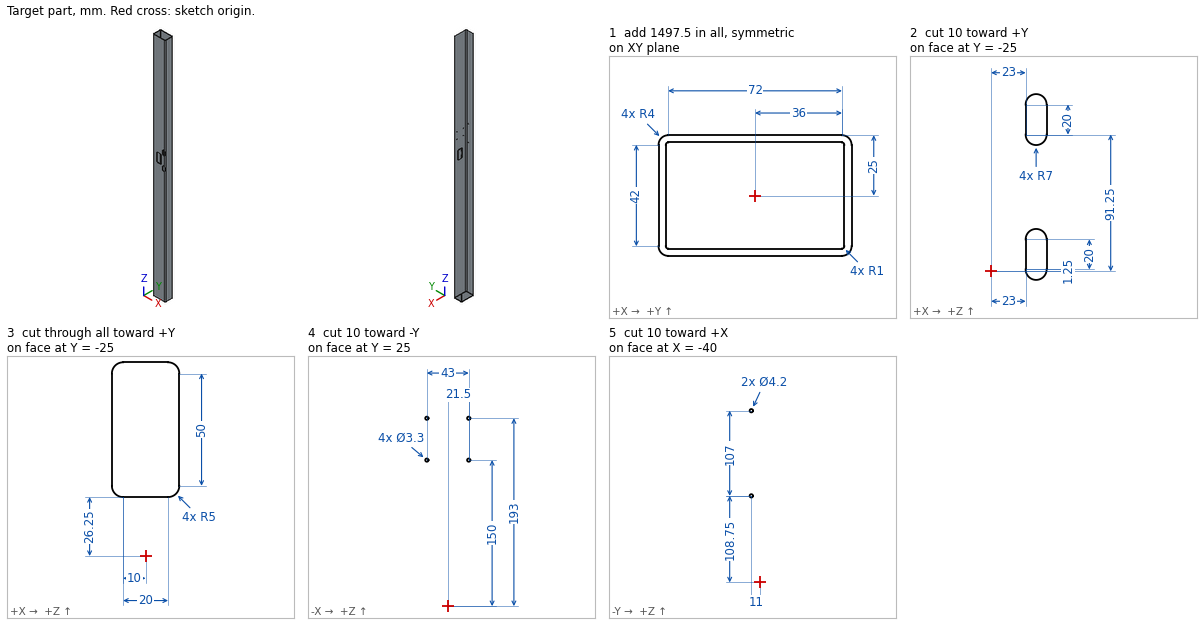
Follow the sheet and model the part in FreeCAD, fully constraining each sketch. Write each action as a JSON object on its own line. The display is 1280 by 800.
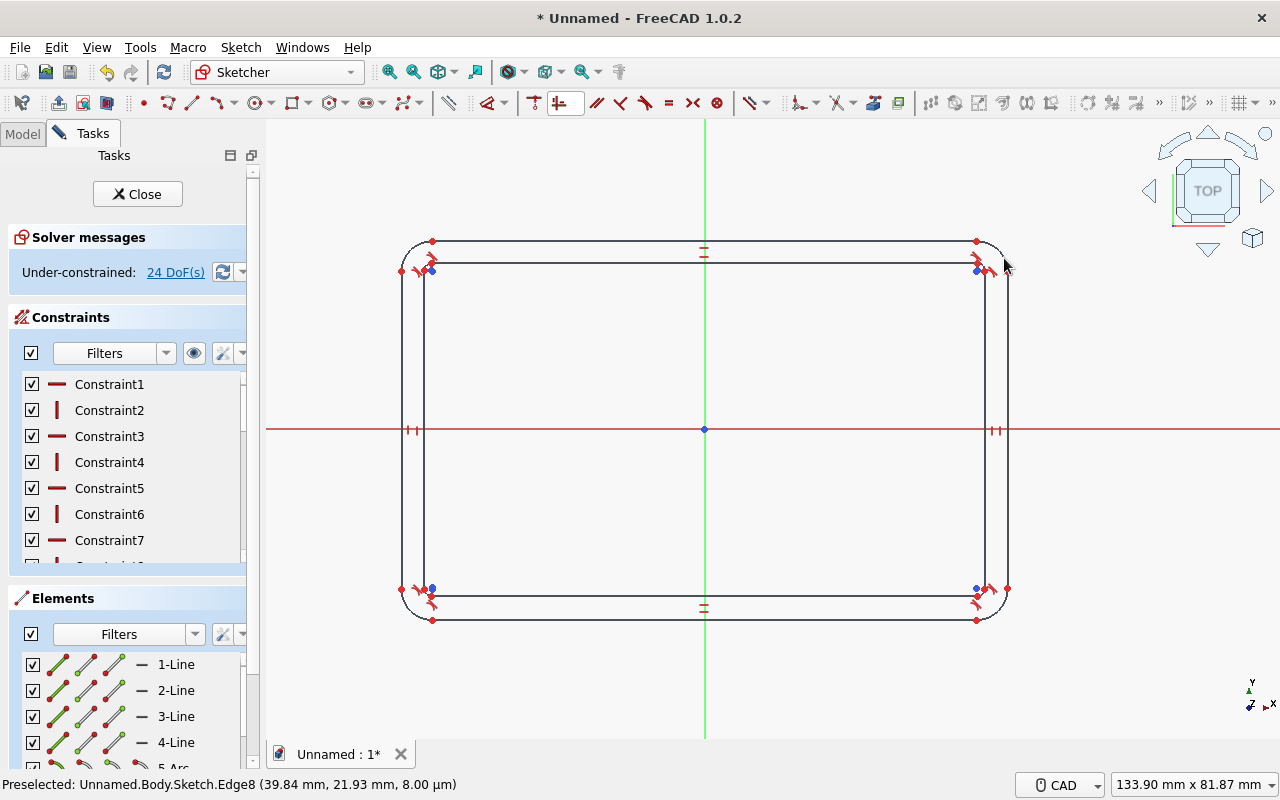
{"action": "left_click", "coordinate": [595, 263]}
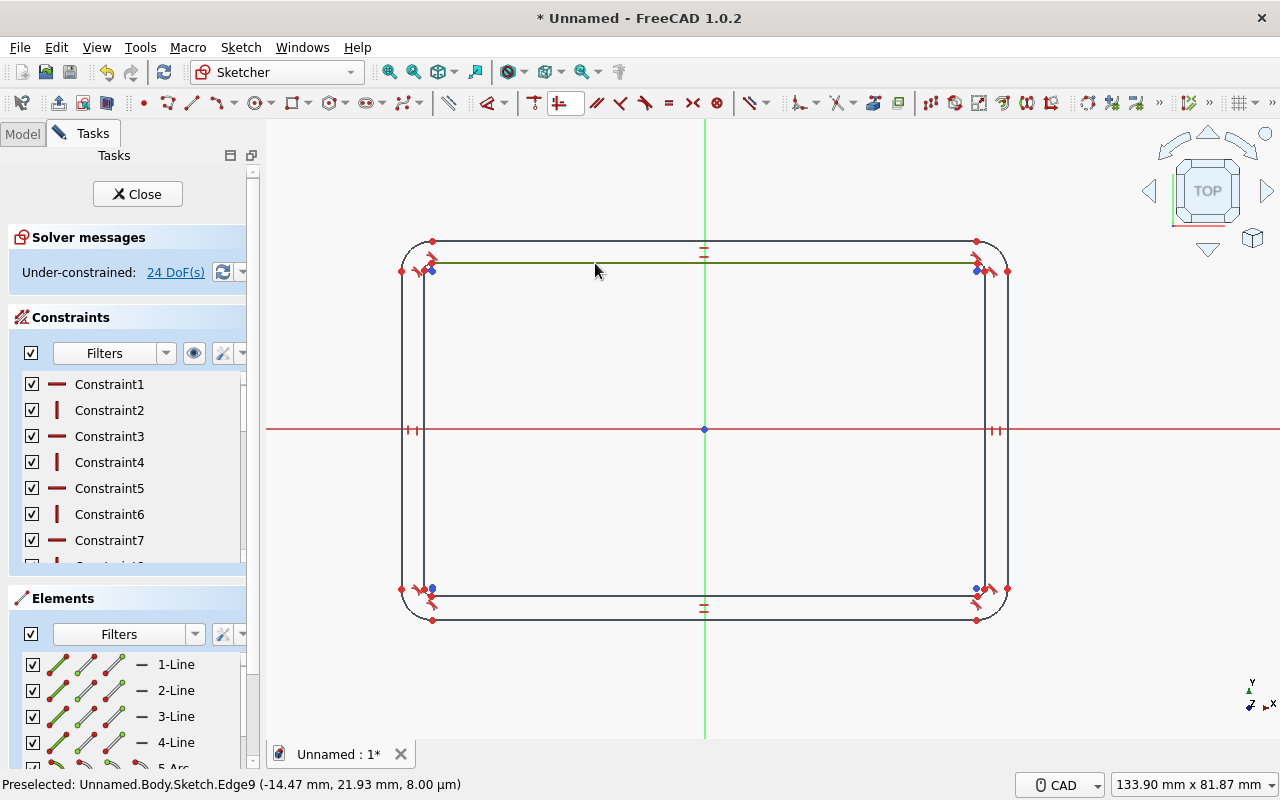
{"action": "scroll", "coordinate": [983, 265], "scroll_direction": "up", "scroll_amount": 5}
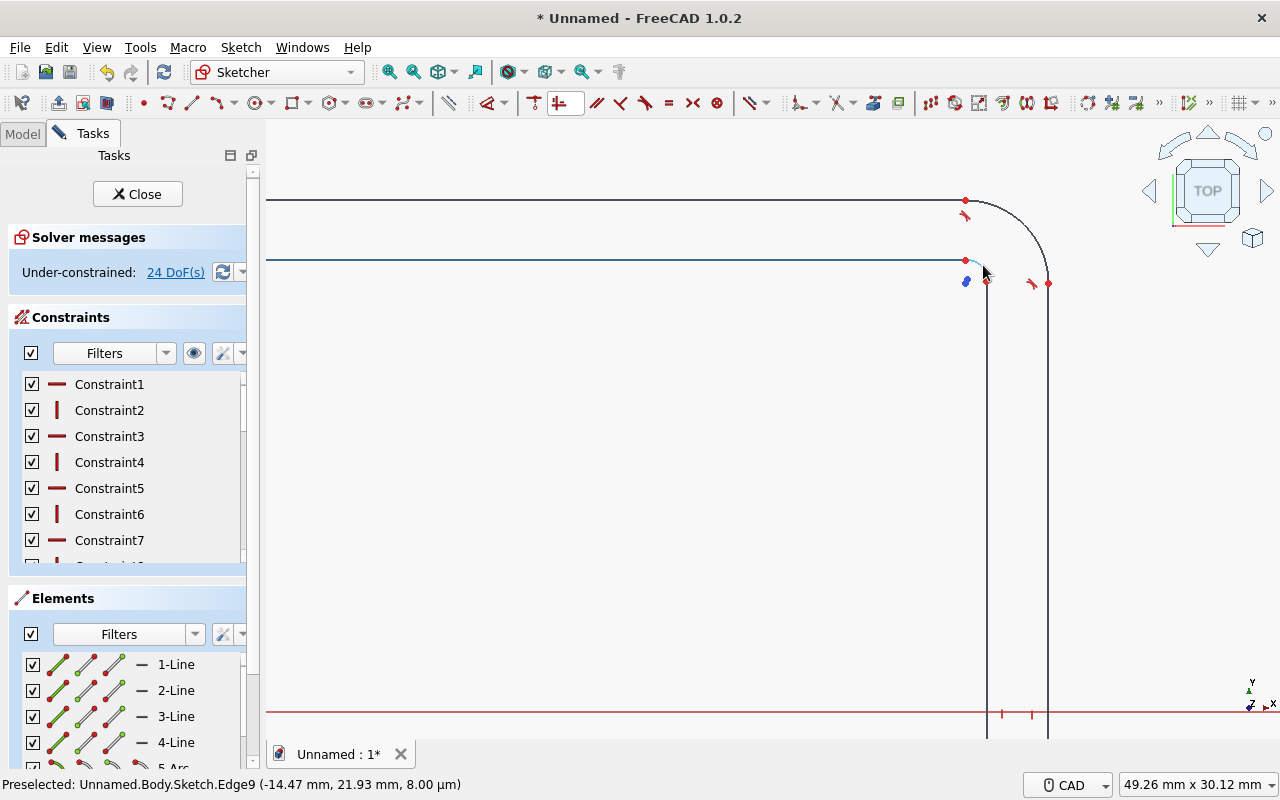
{"action": "left_click", "coordinate": [981, 266]}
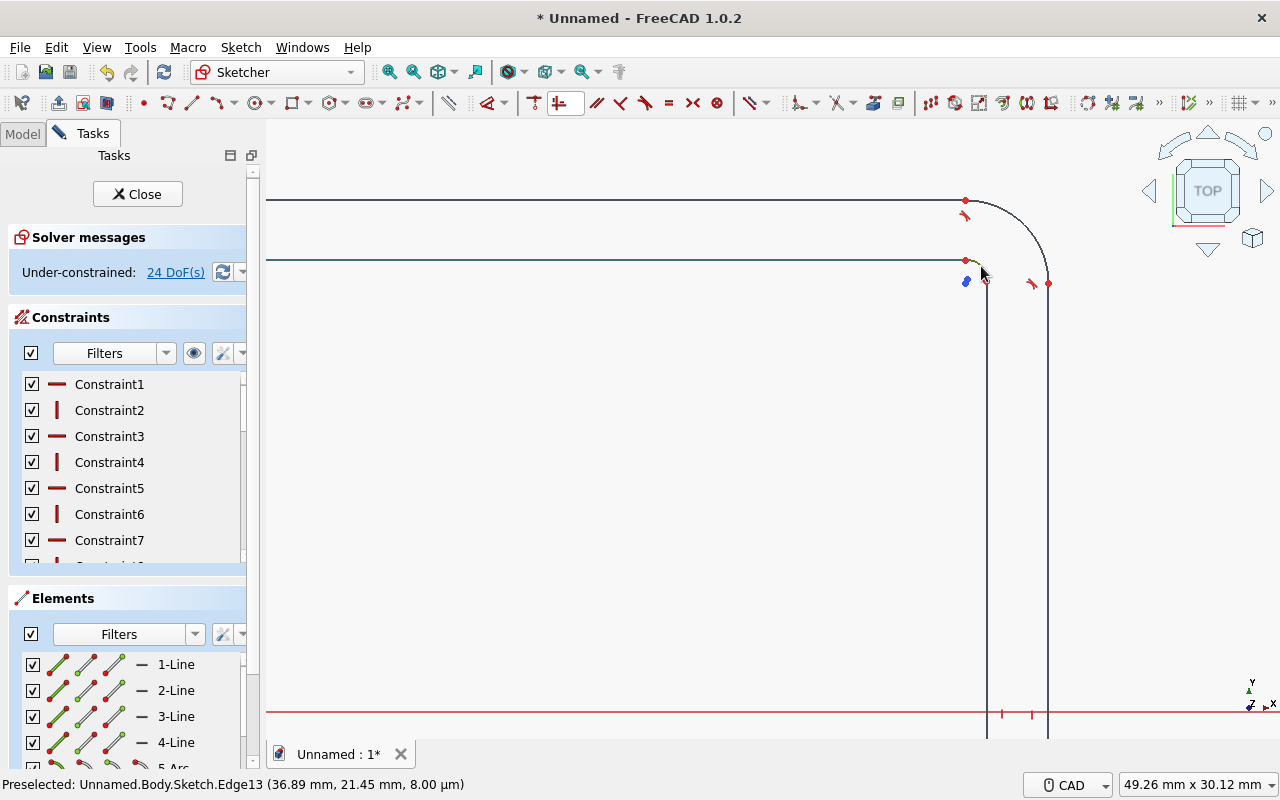
{"action": "key", "text": "t"}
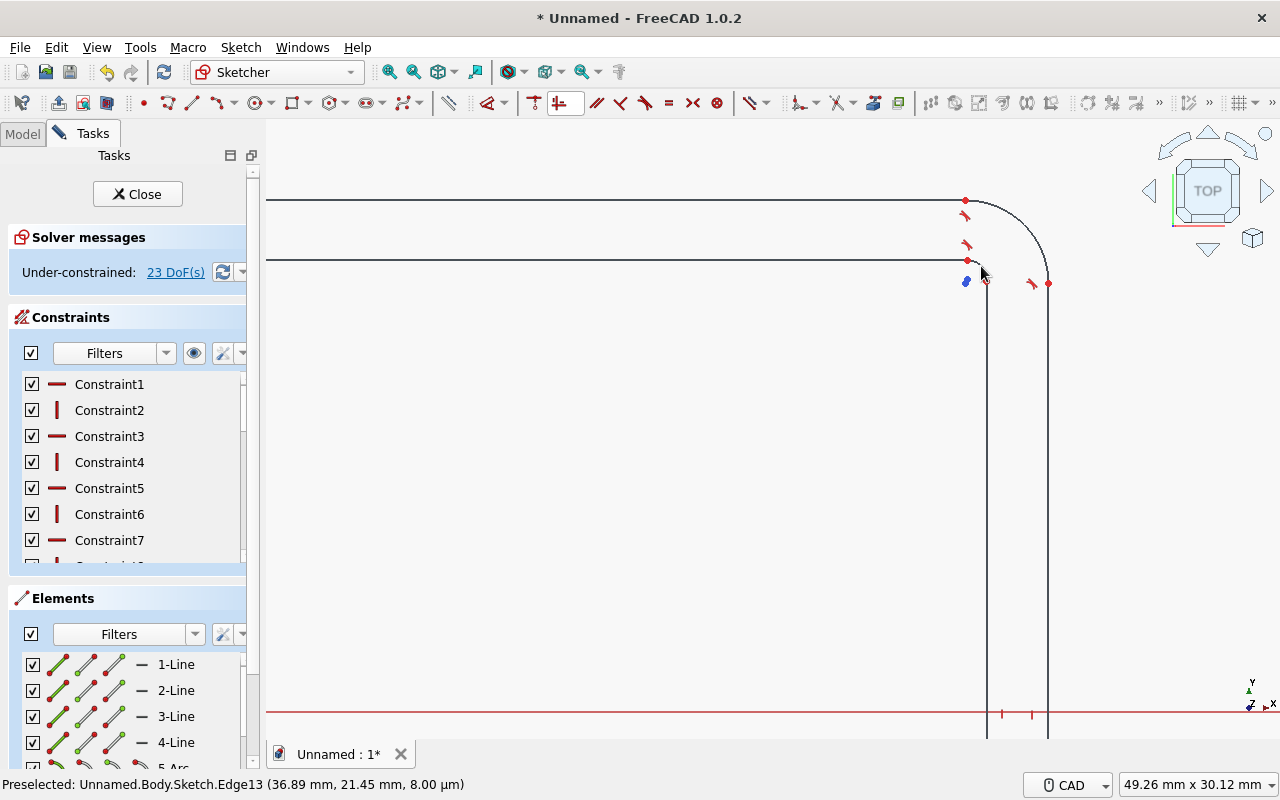
{"action": "left_click", "coordinate": [523, 260]}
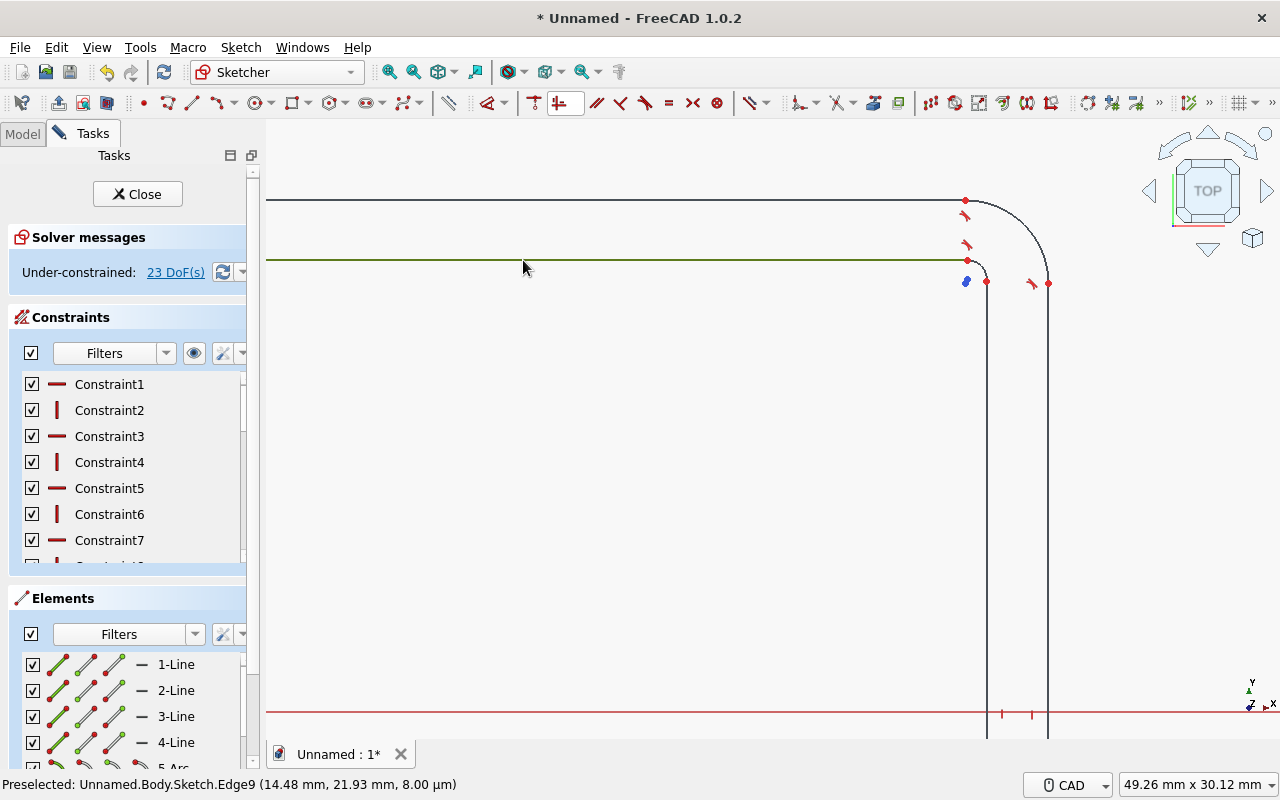
{"action": "scroll", "coordinate": [984, 264], "scroll_direction": "down", "scroll_amount": 5}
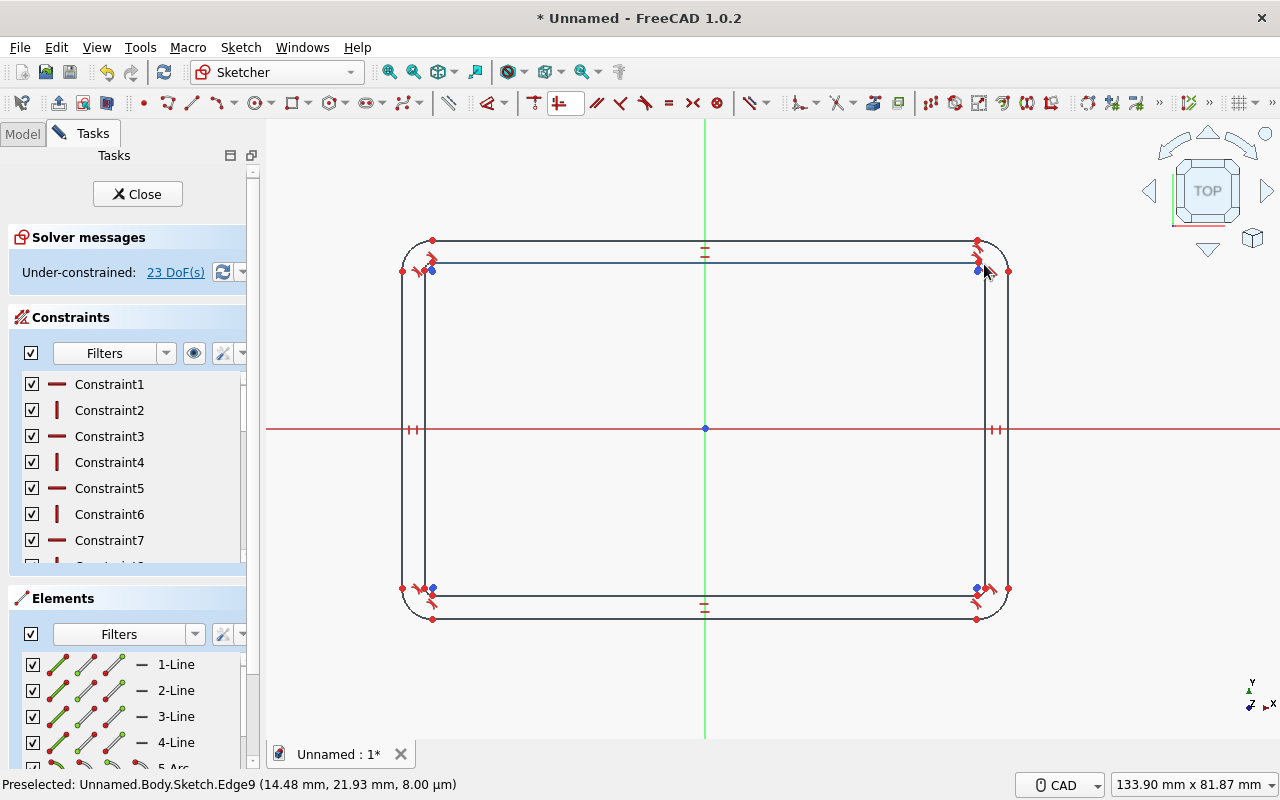
{"action": "scroll", "coordinate": [429, 263], "scroll_direction": "up", "scroll_amount": 7}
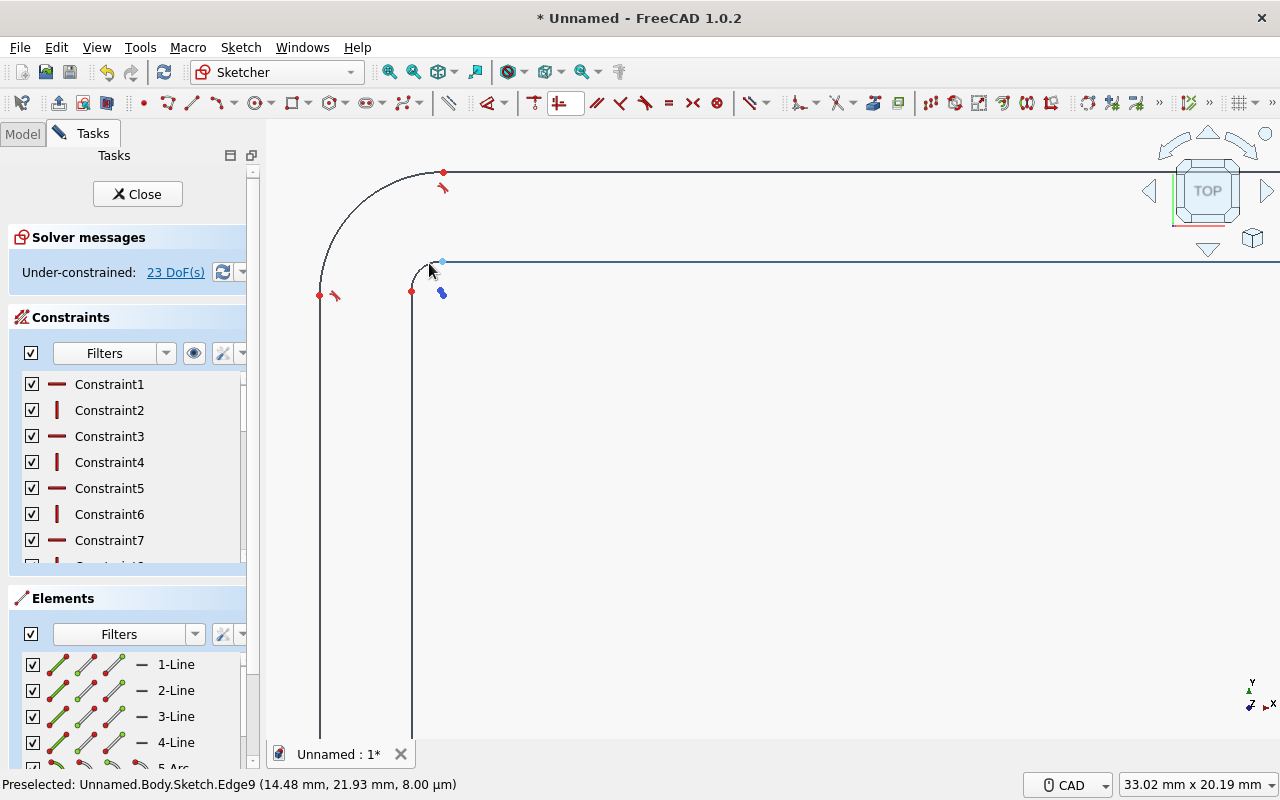
{"action": "left_click", "coordinate": [428, 264]}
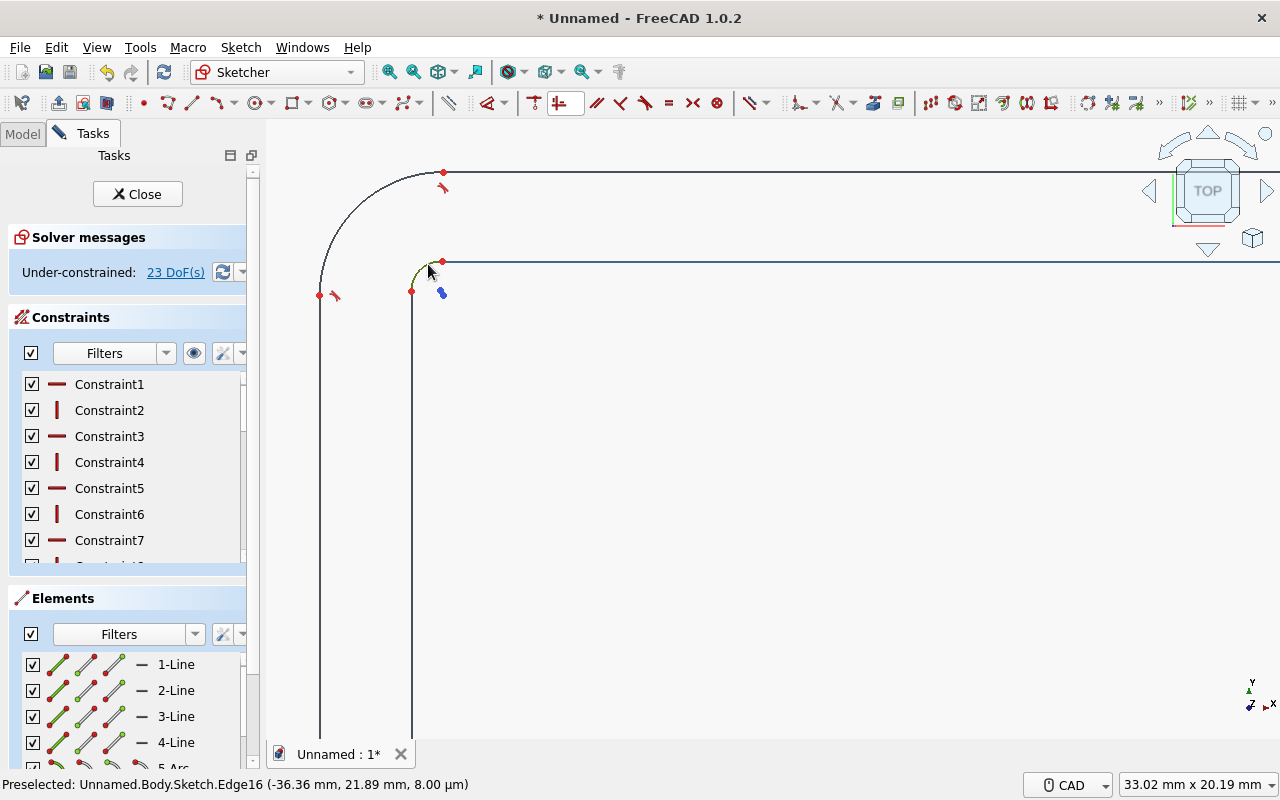
{"action": "key", "text": "t"}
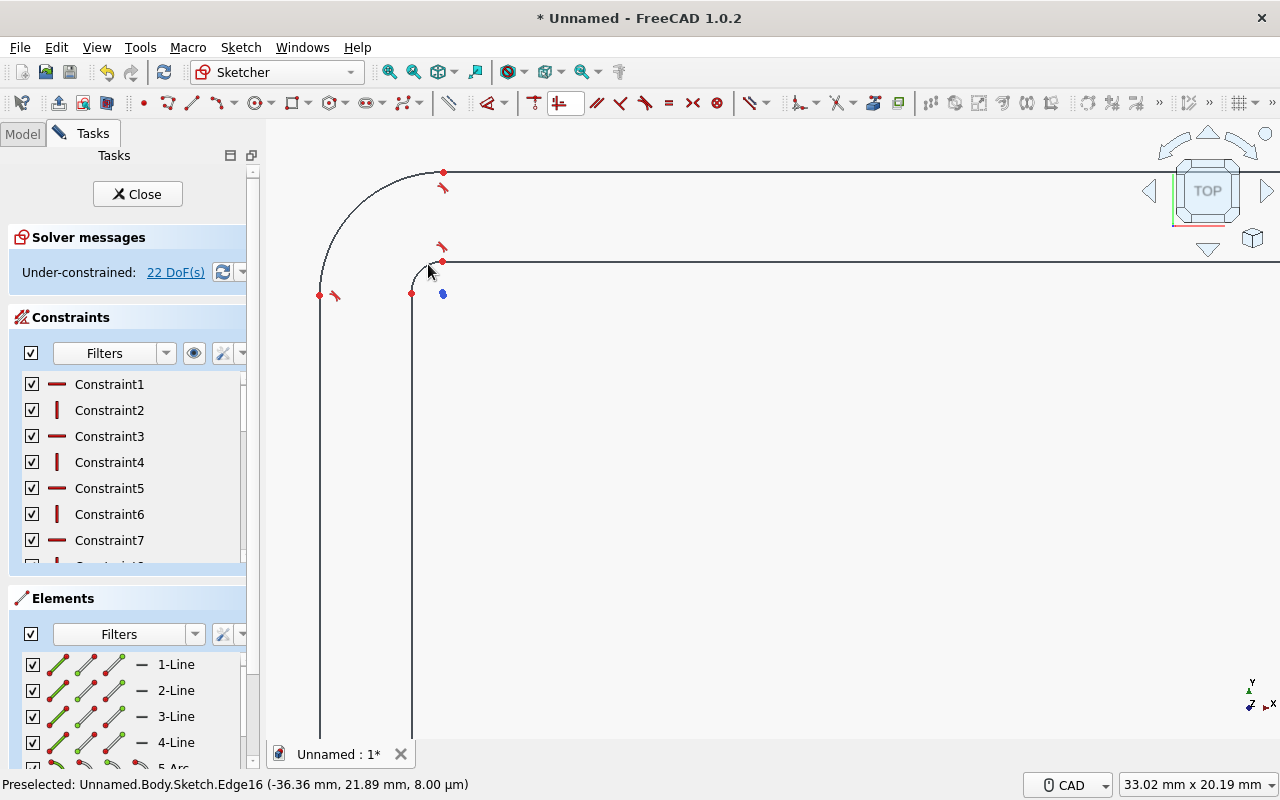
{"action": "scroll", "coordinate": [428, 263], "scroll_direction": "down", "scroll_amount": 7}